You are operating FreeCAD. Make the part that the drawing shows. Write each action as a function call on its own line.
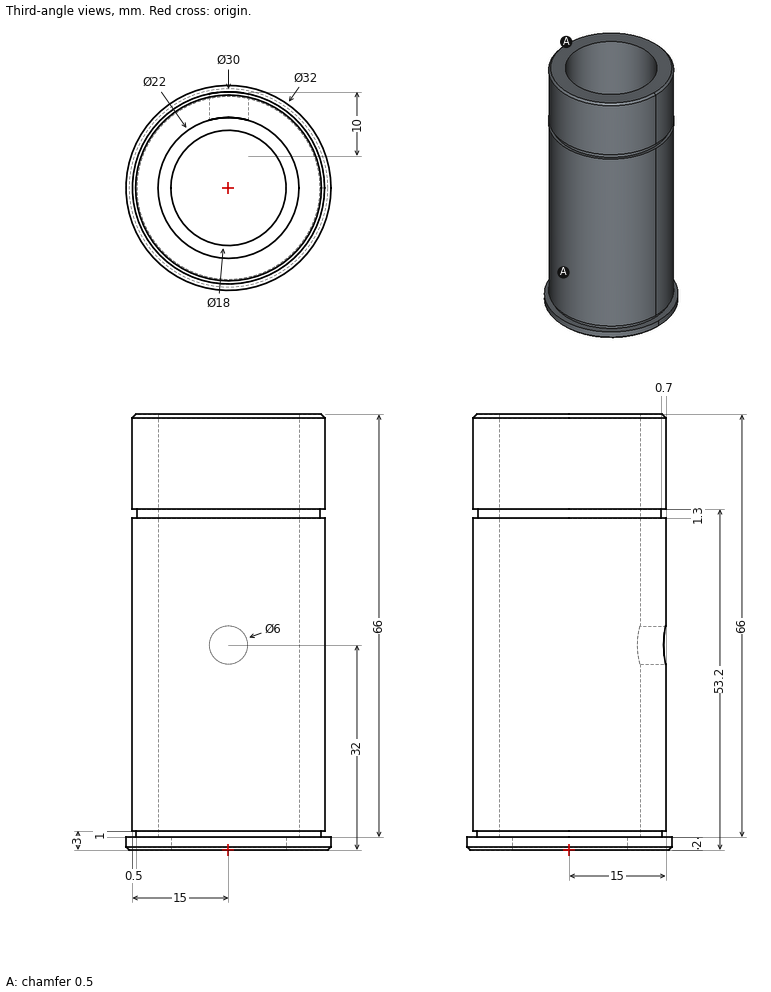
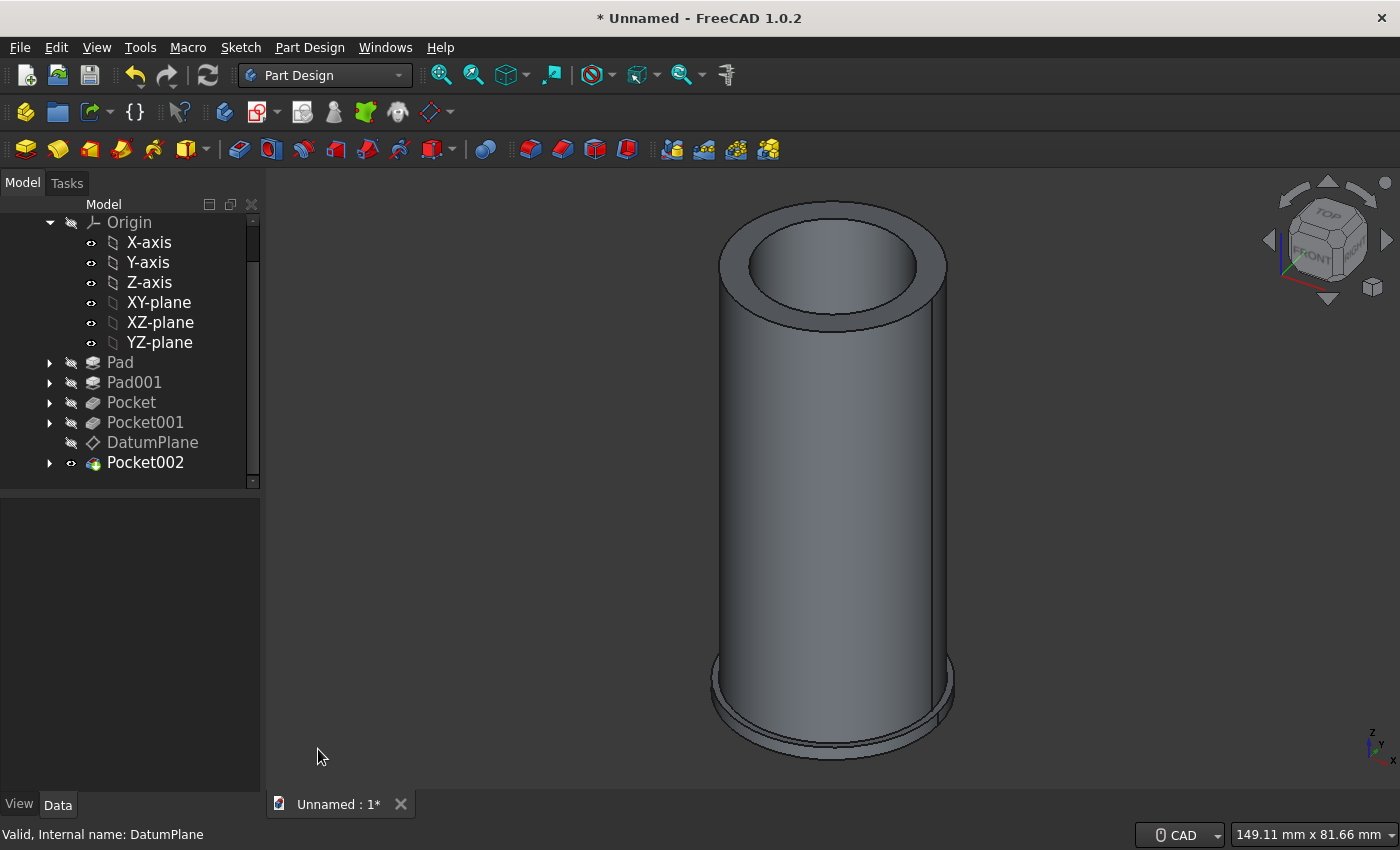
click(258, 112)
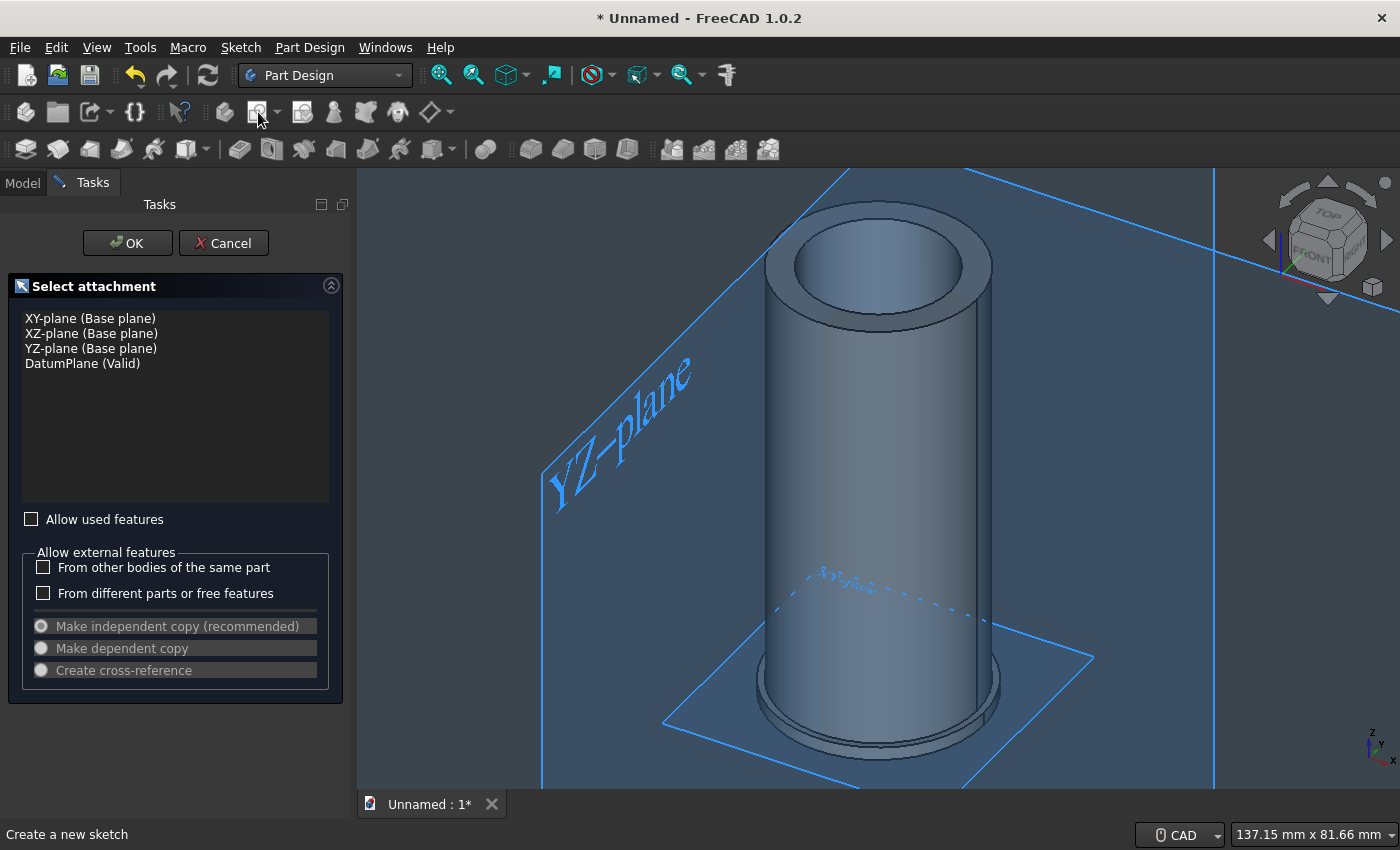
click(82, 348)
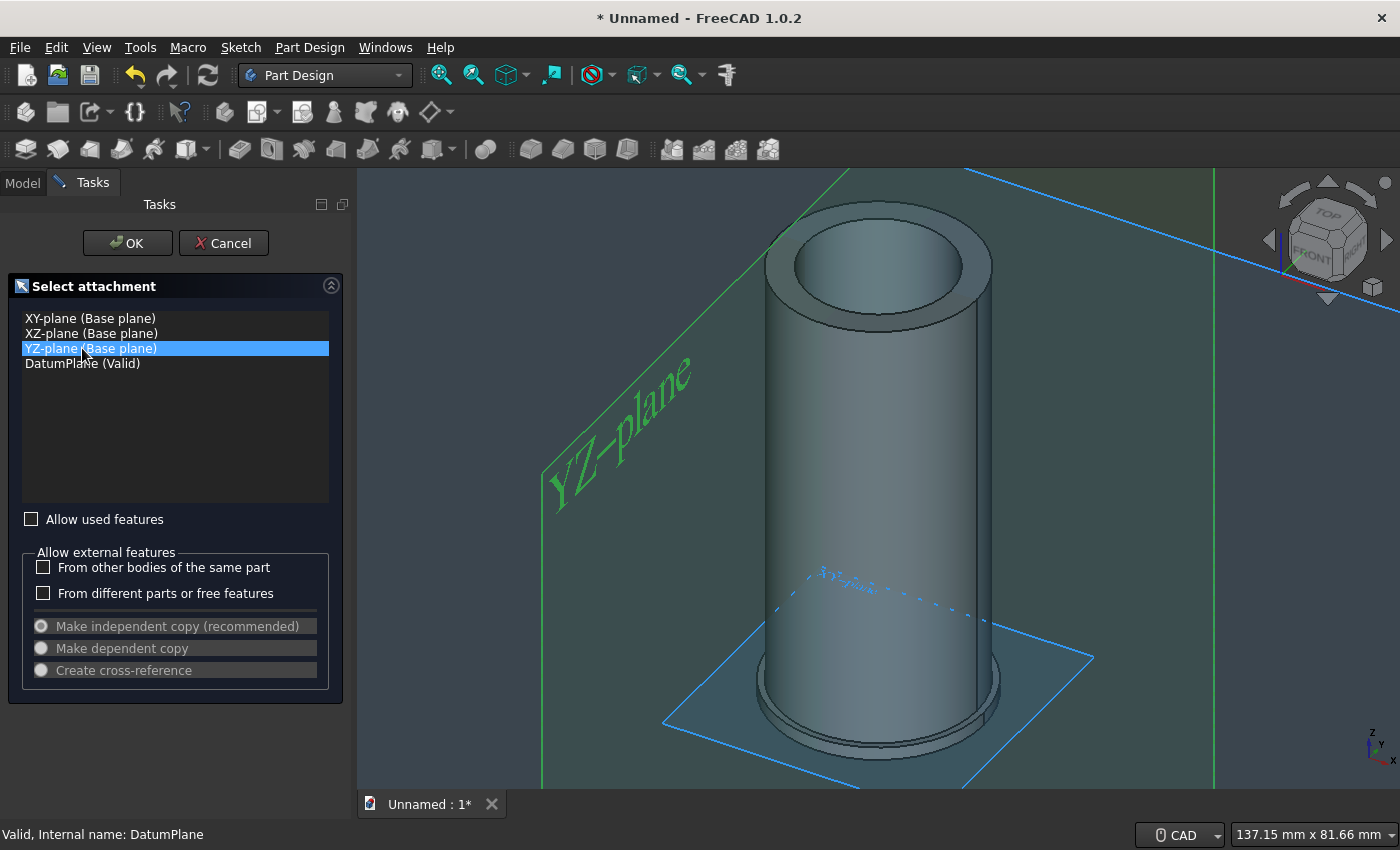
click(128, 243)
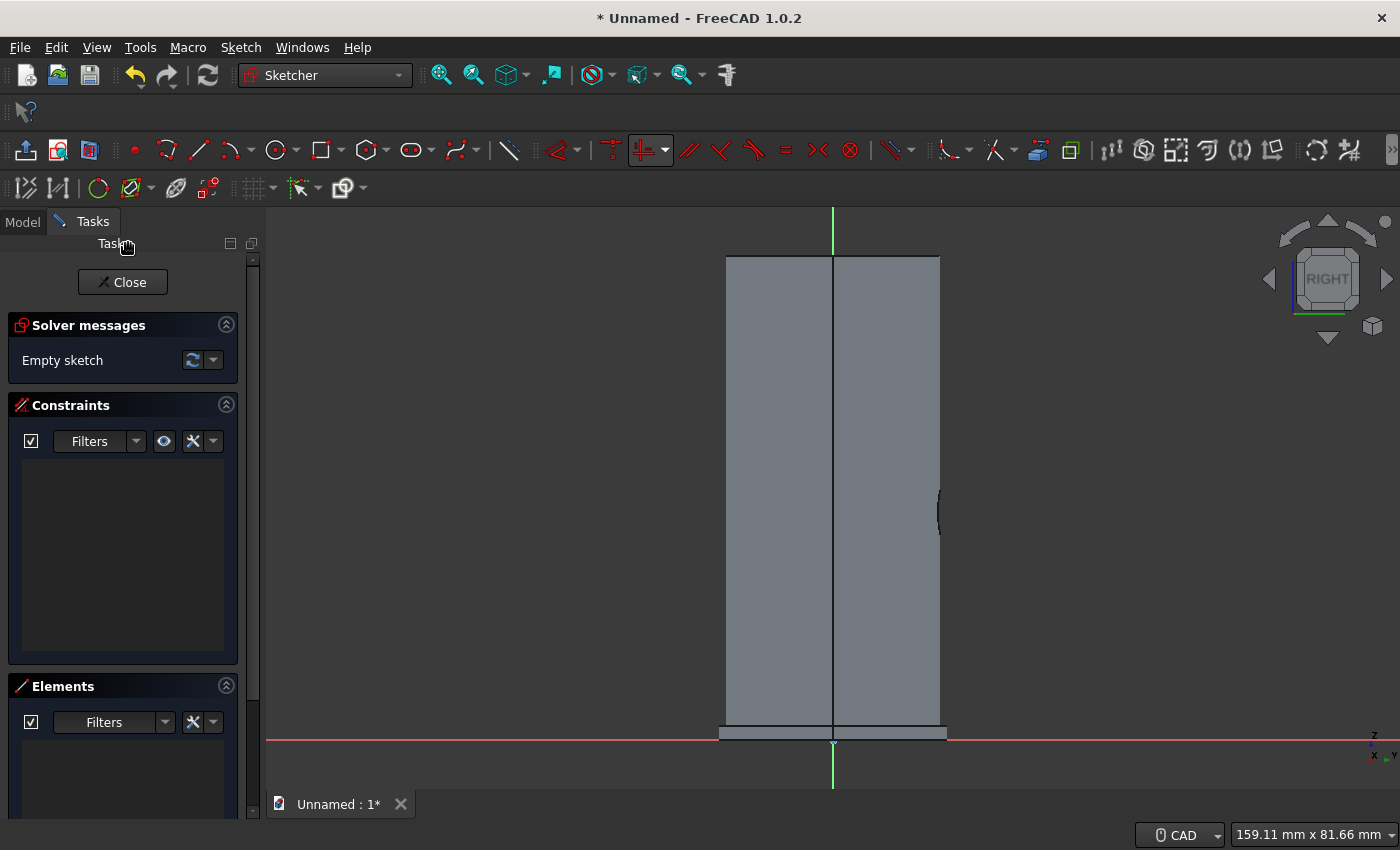
click(90, 150)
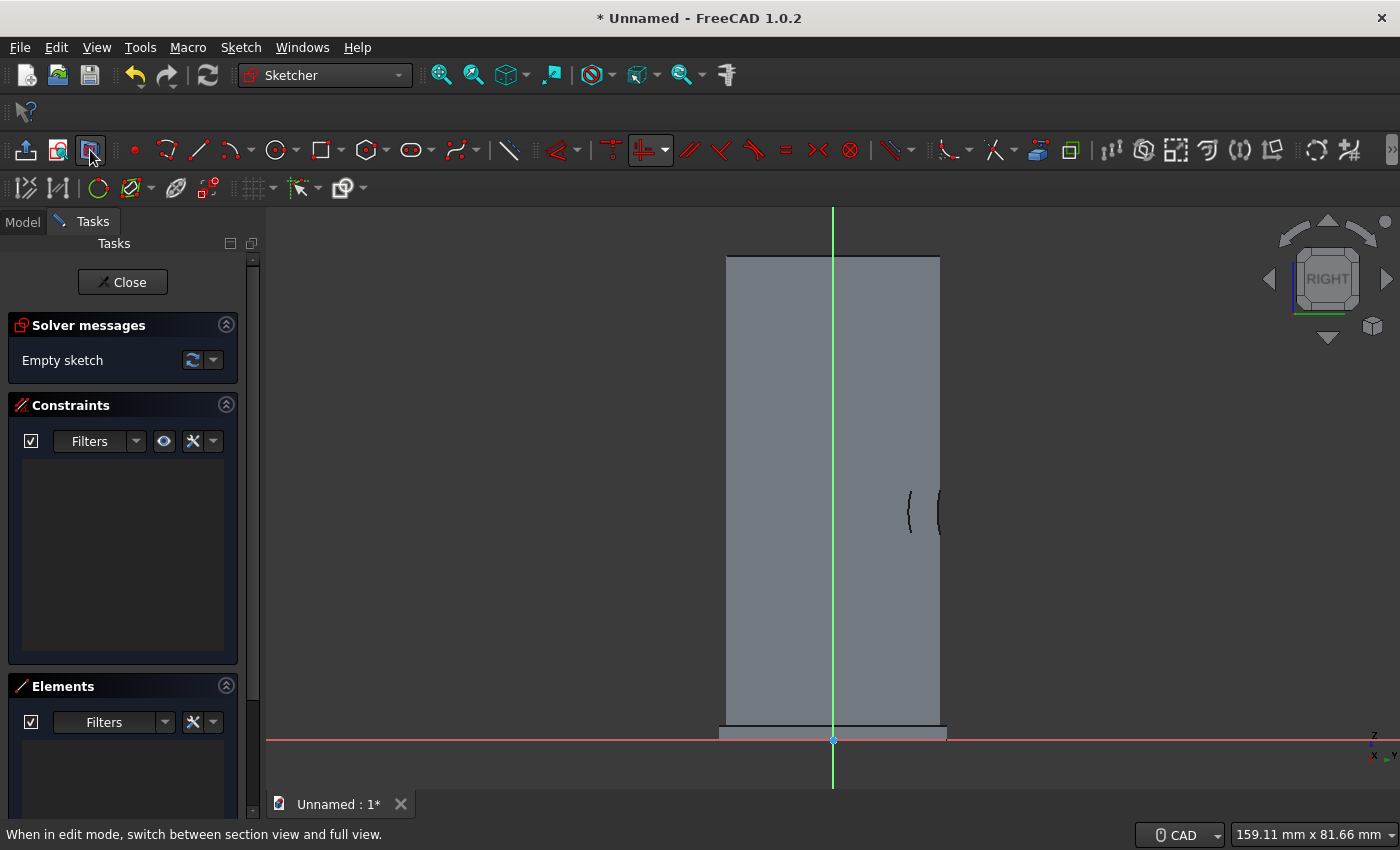
scroll(946, 359, up, 15)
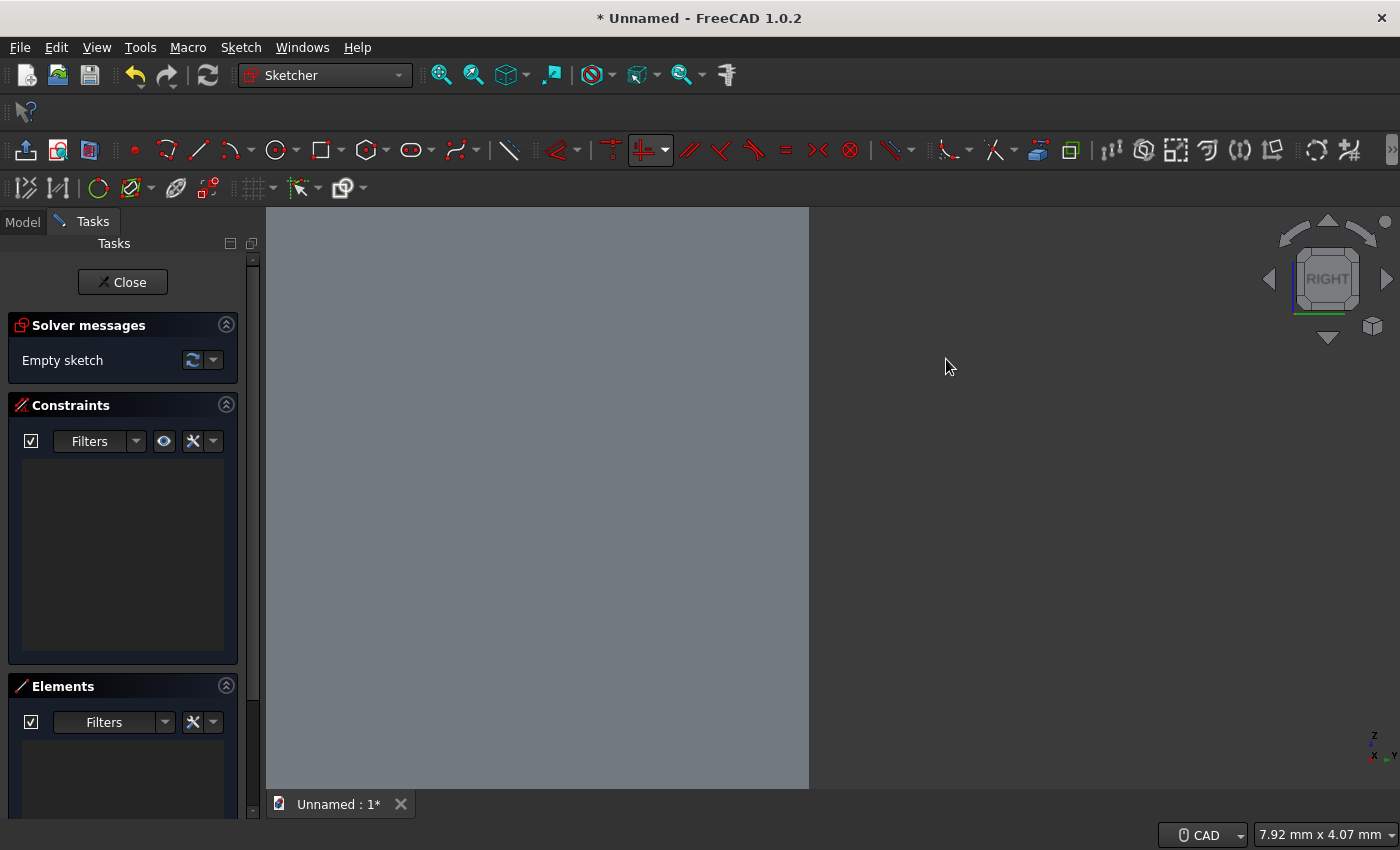
scroll(759, 481, up, 3)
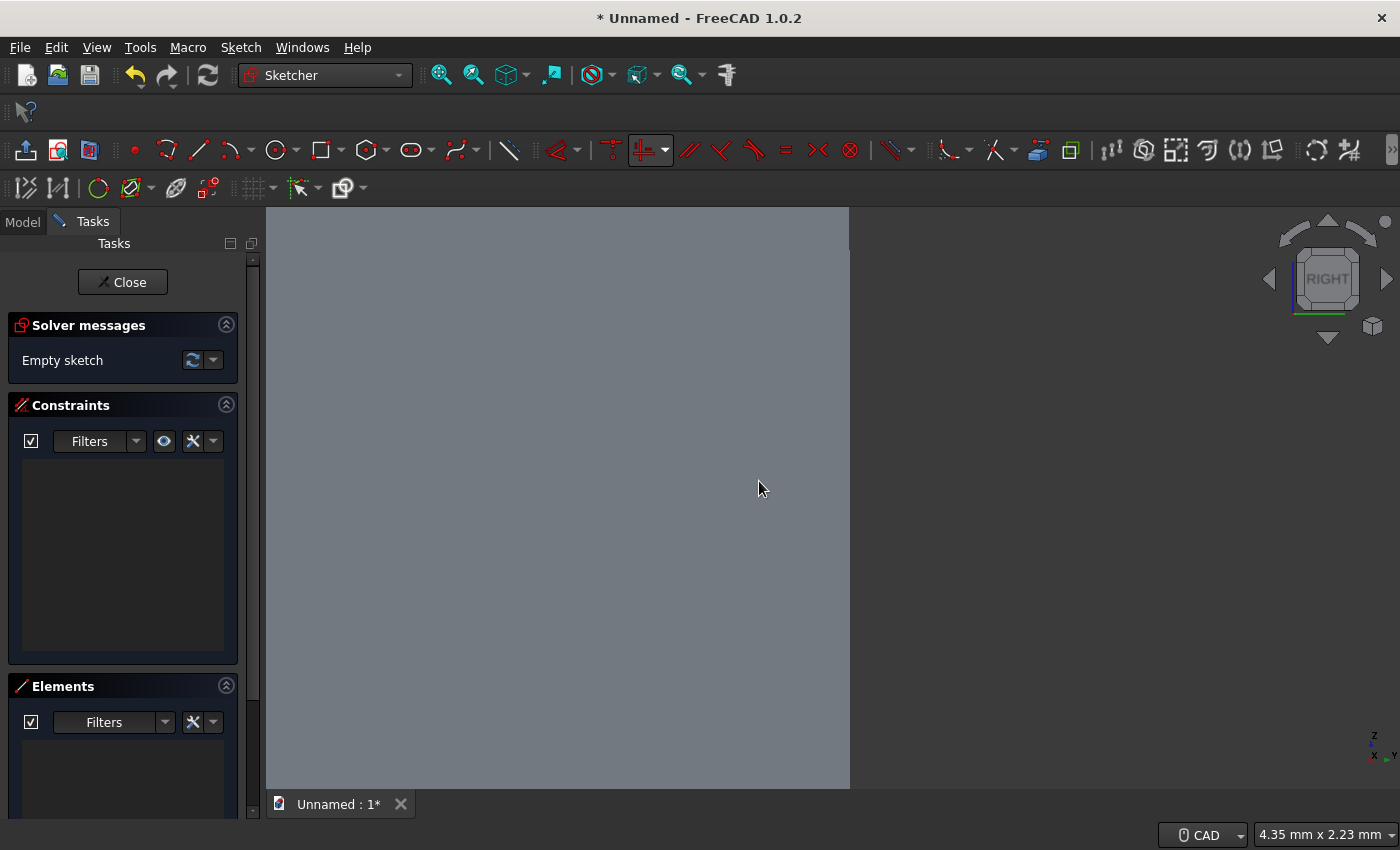
click(322, 150)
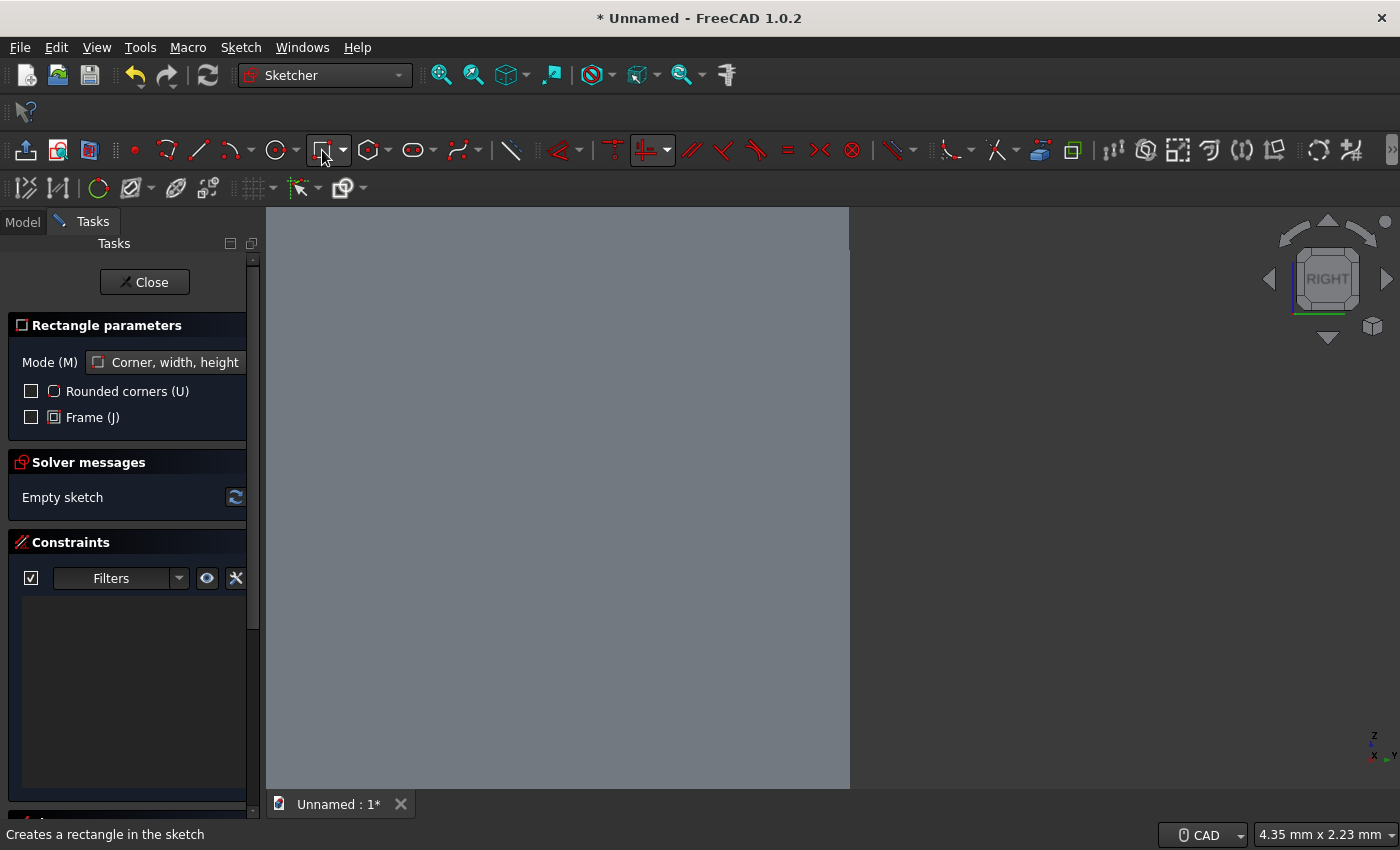
click(673, 328)
move(856, 667)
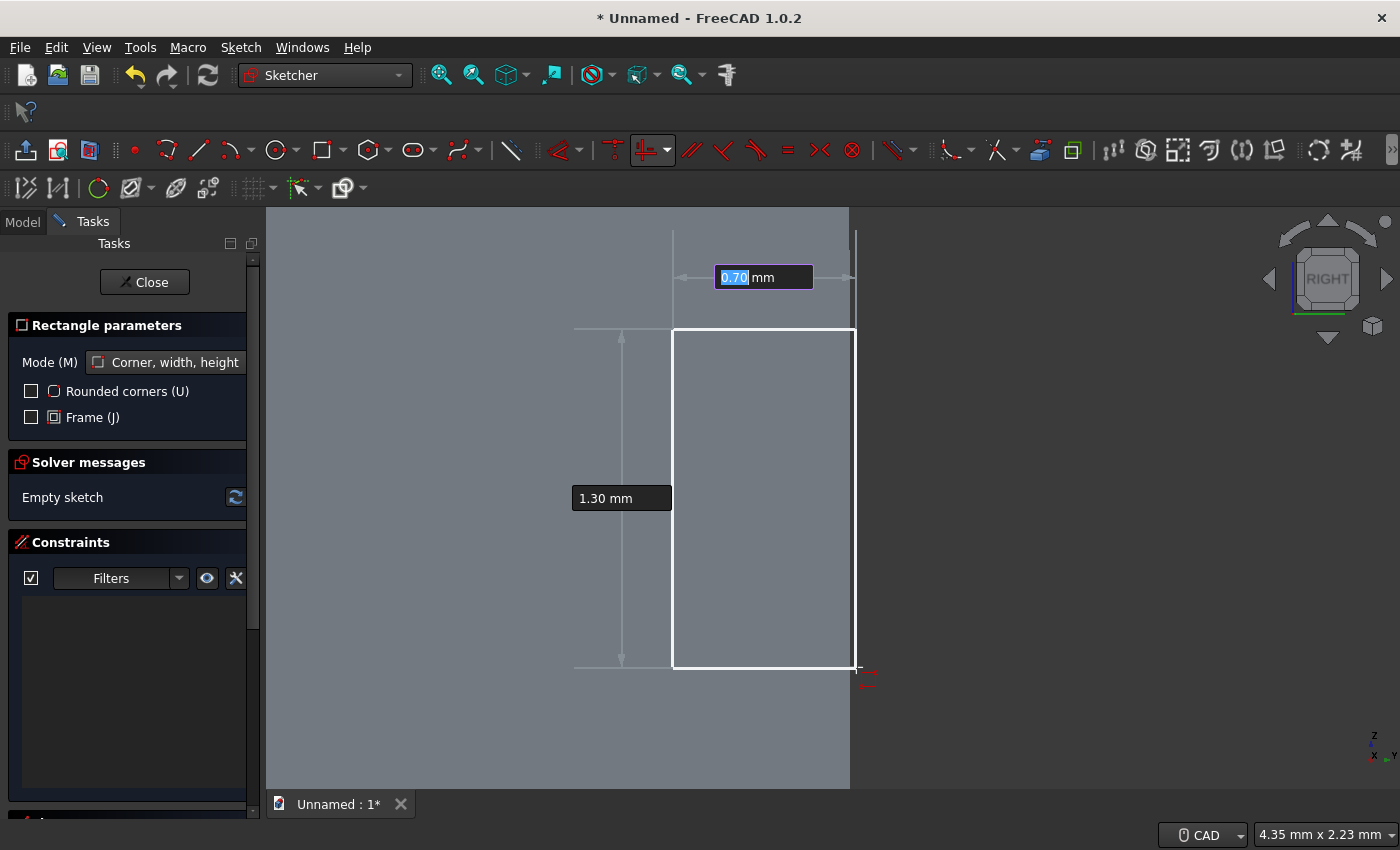
text(0.7)
key(Tab)
text(1.3)
key(Return)
key(Escape)